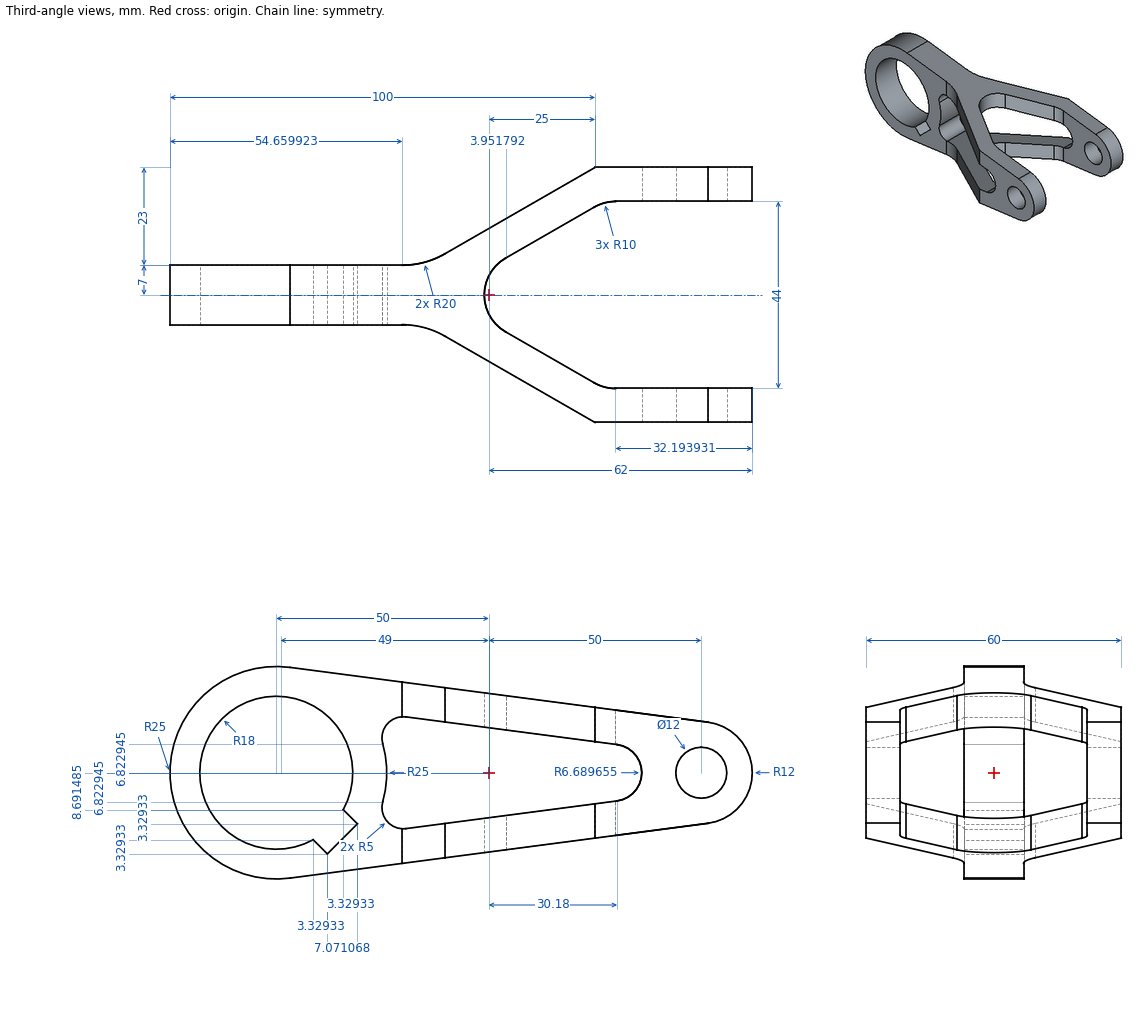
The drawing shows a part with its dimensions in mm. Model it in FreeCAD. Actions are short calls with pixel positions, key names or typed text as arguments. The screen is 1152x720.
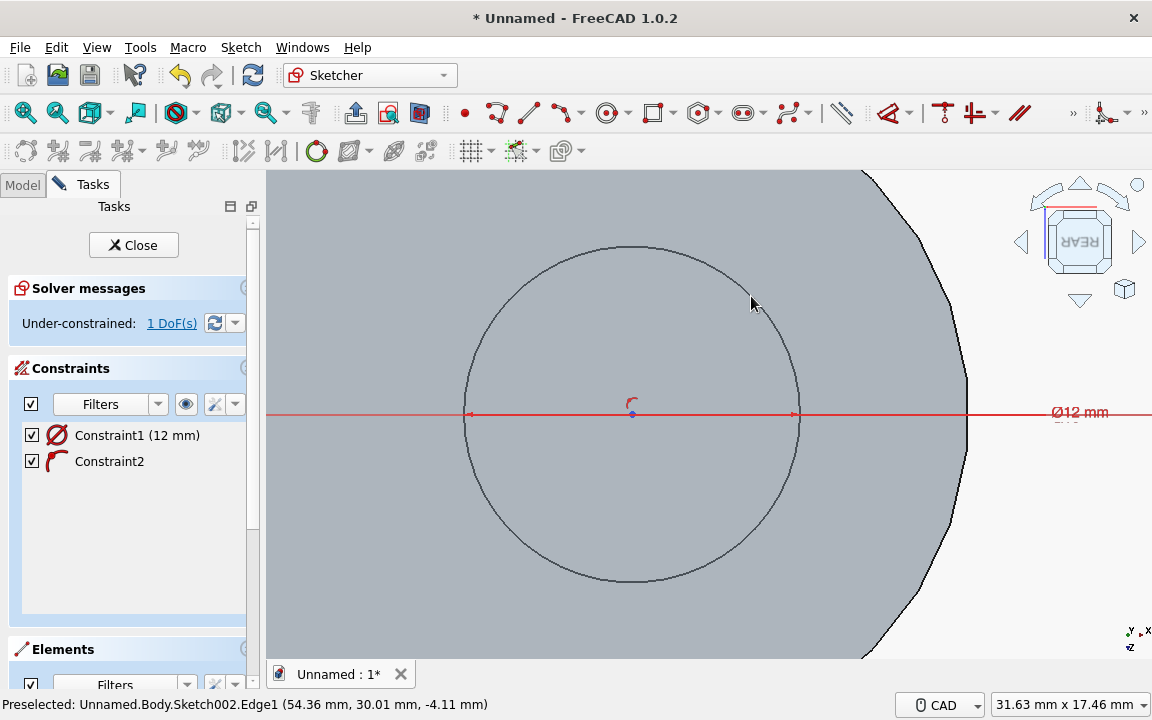
click(888, 114)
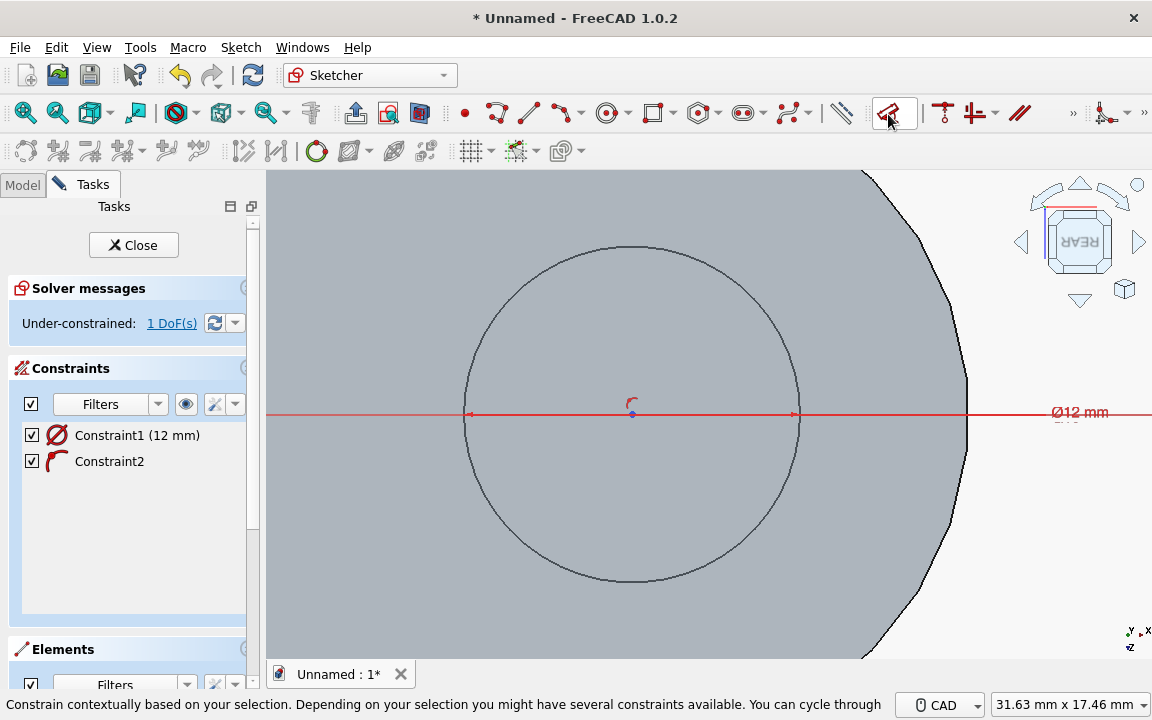
click(632, 414)
click(385, 448)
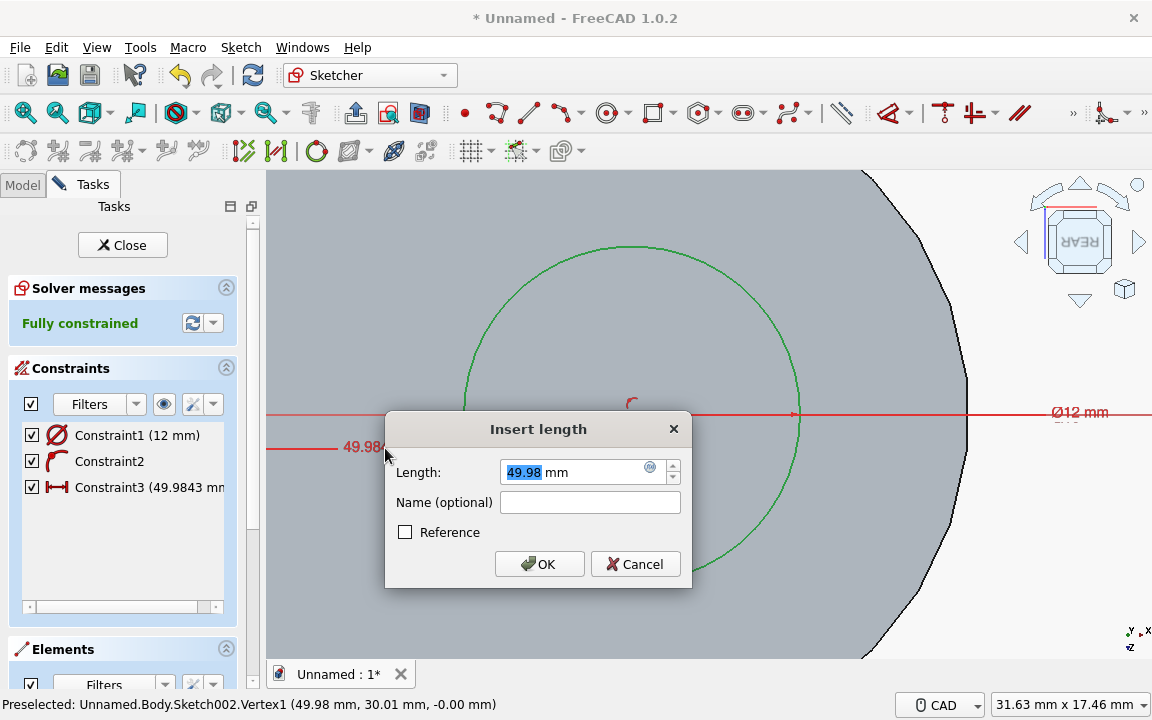
text(50)
key(Return)
key(Escape)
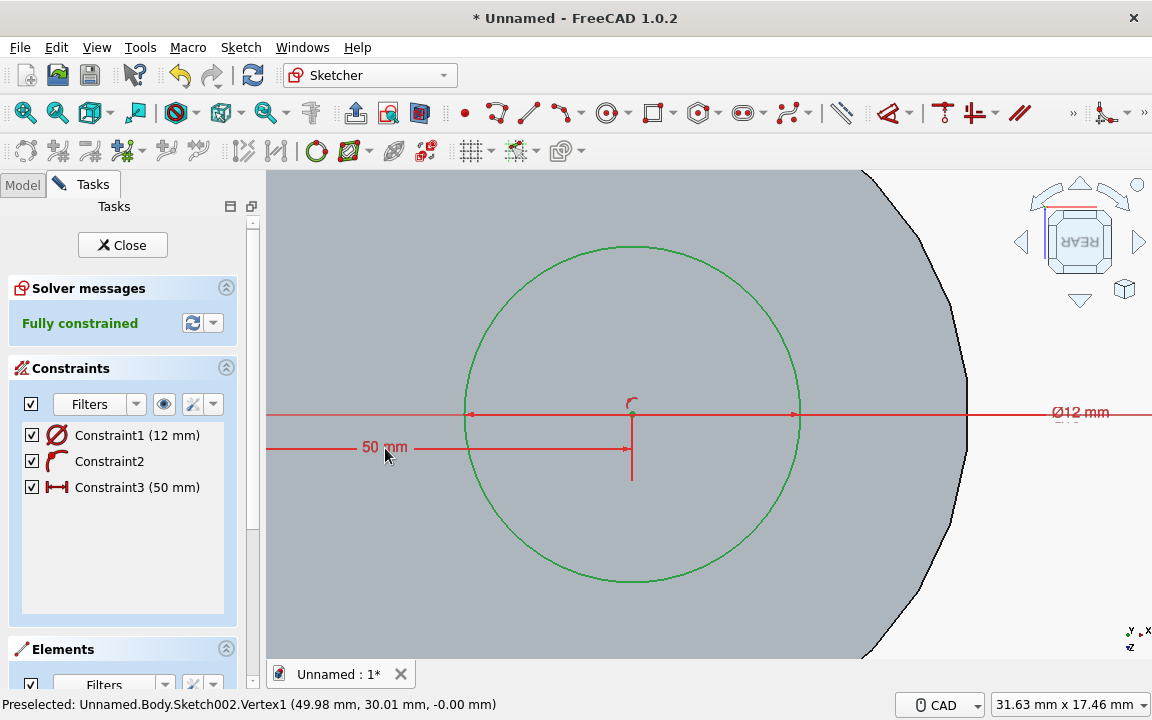
click(123, 245)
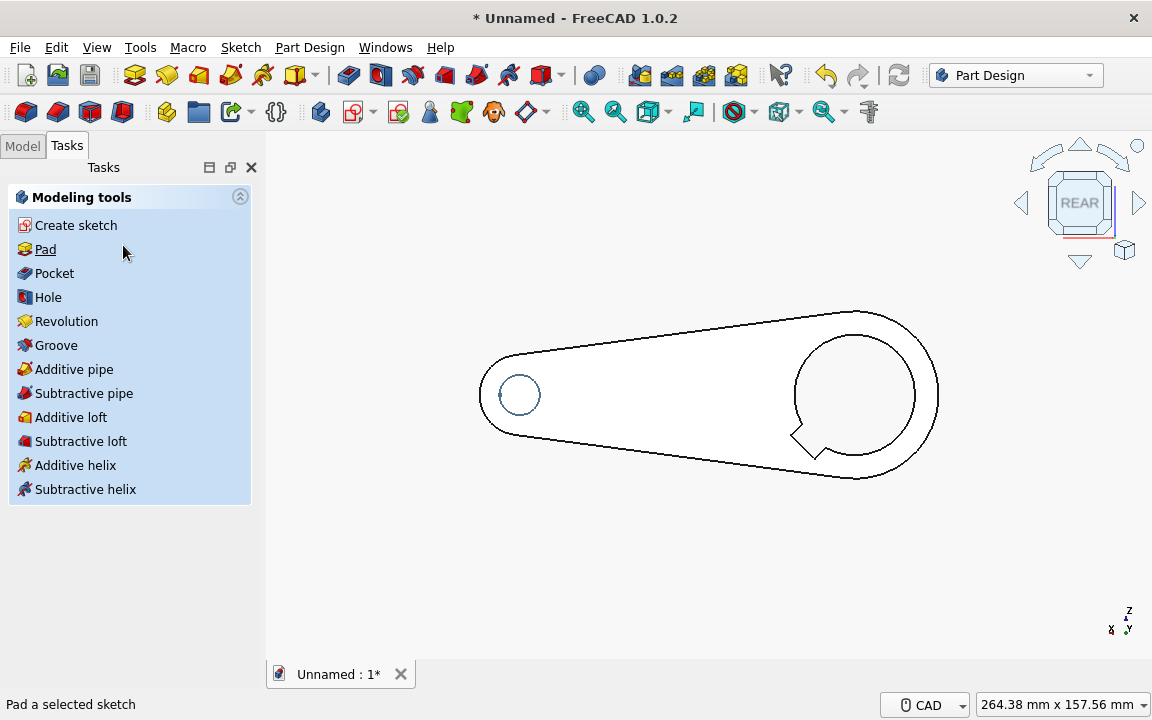
click(350, 76)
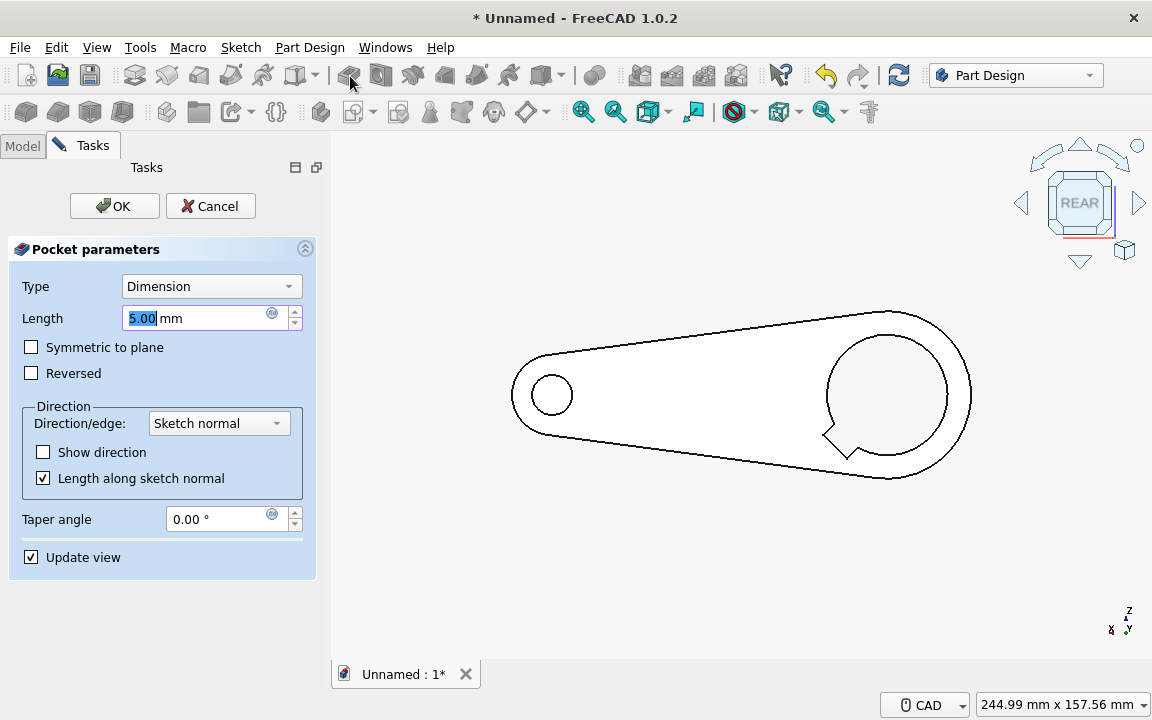
click(212, 286)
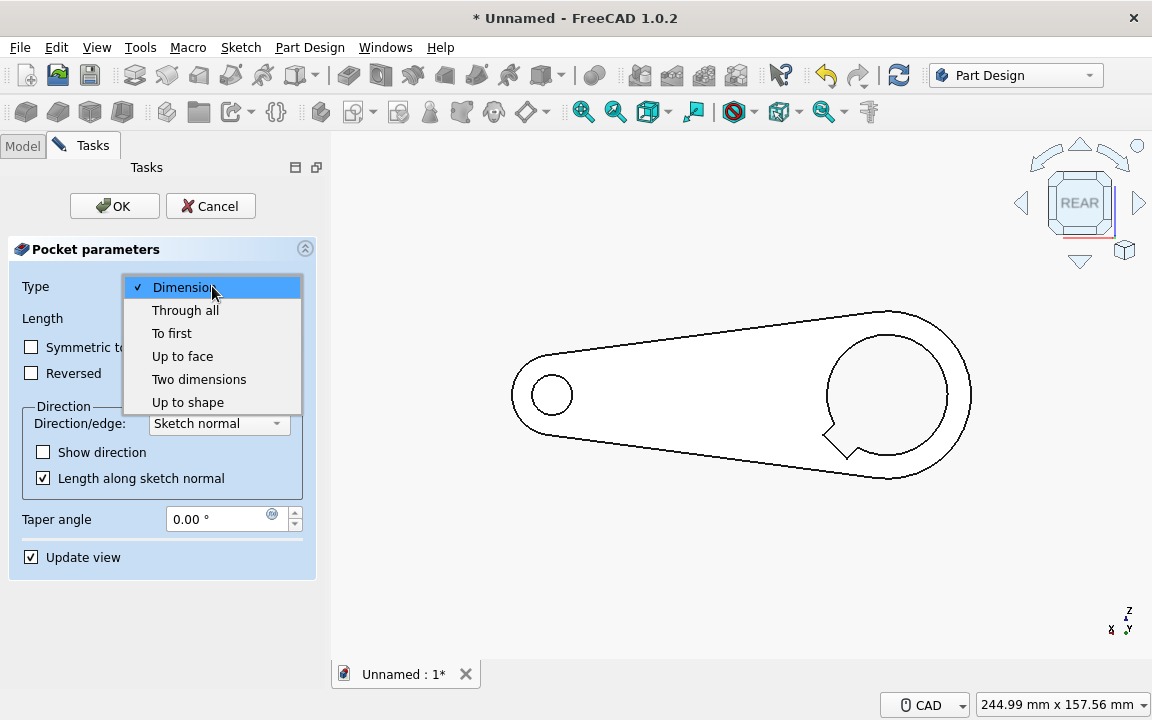
click(212, 310)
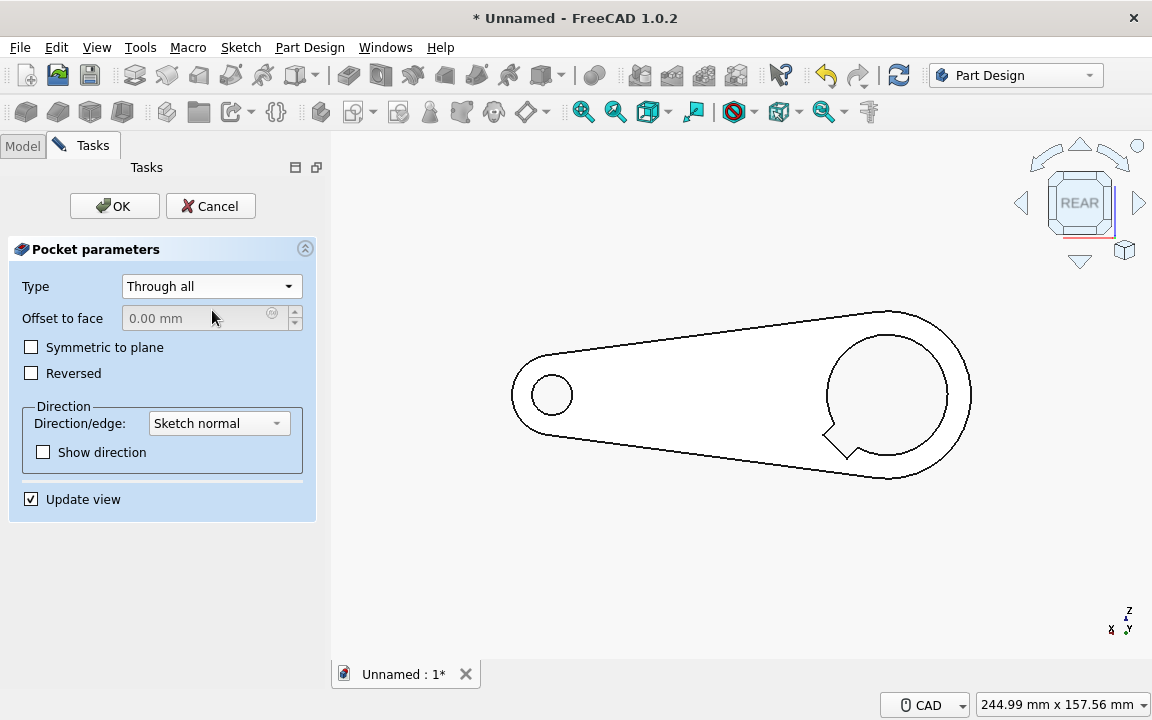
click(115, 206)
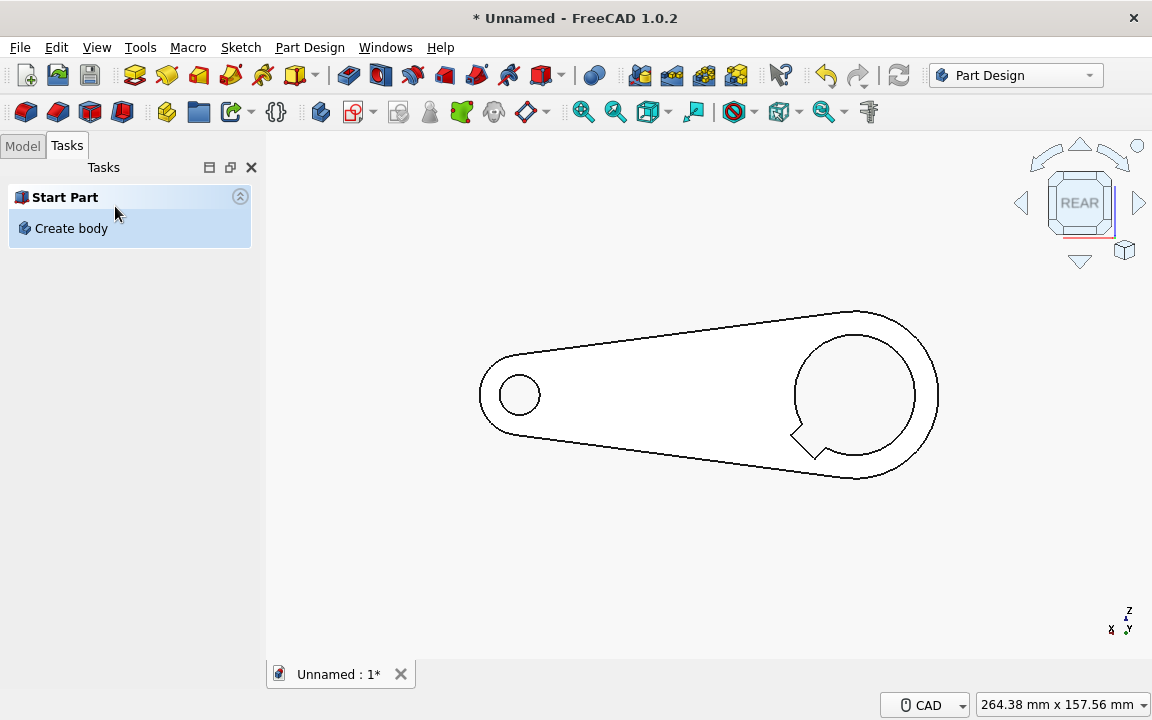
click(709, 394)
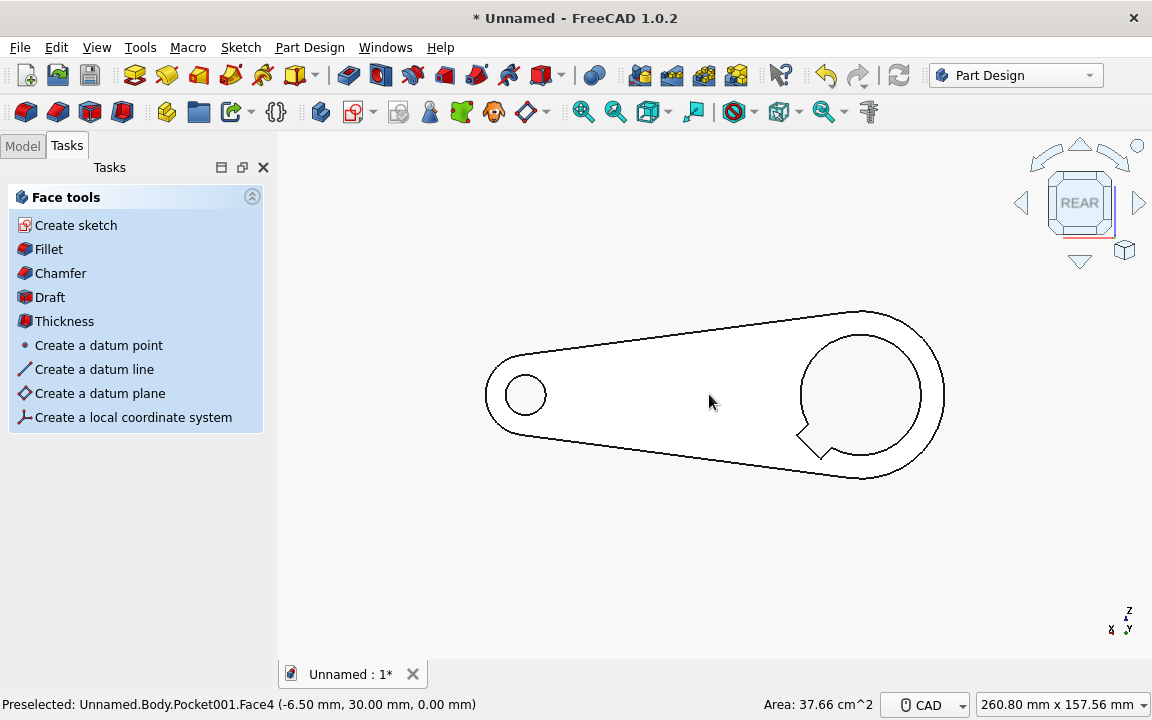
click(354, 112)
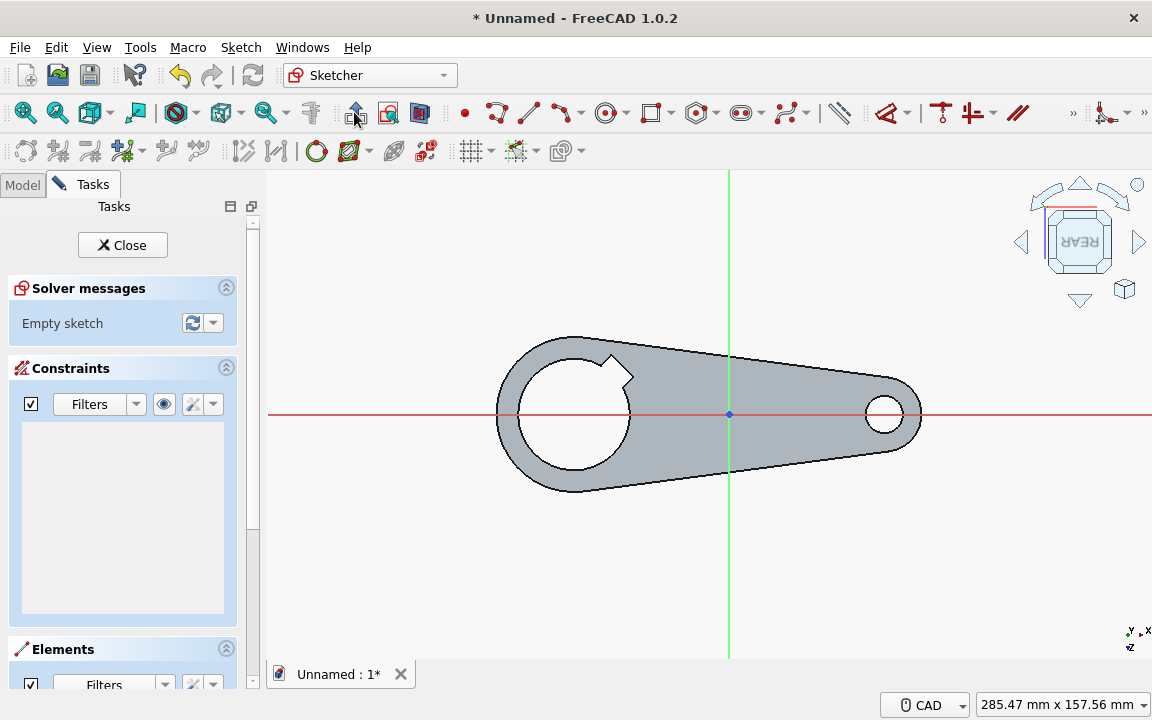
scroll(808, 414, up, 5)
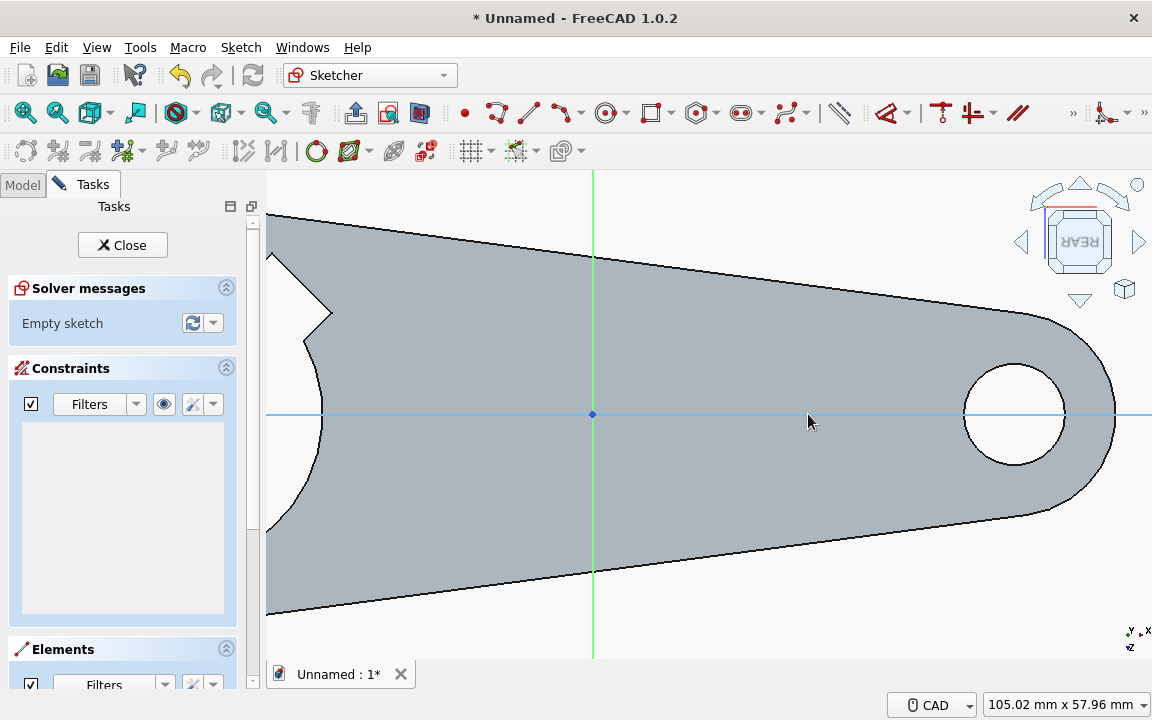
click(530, 114)